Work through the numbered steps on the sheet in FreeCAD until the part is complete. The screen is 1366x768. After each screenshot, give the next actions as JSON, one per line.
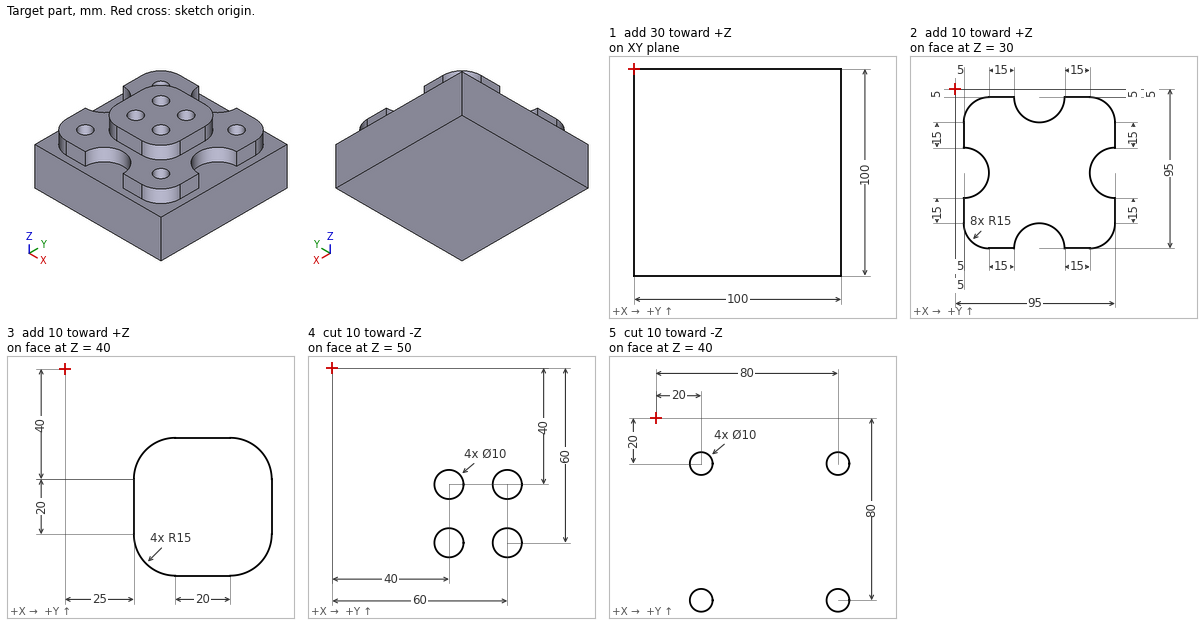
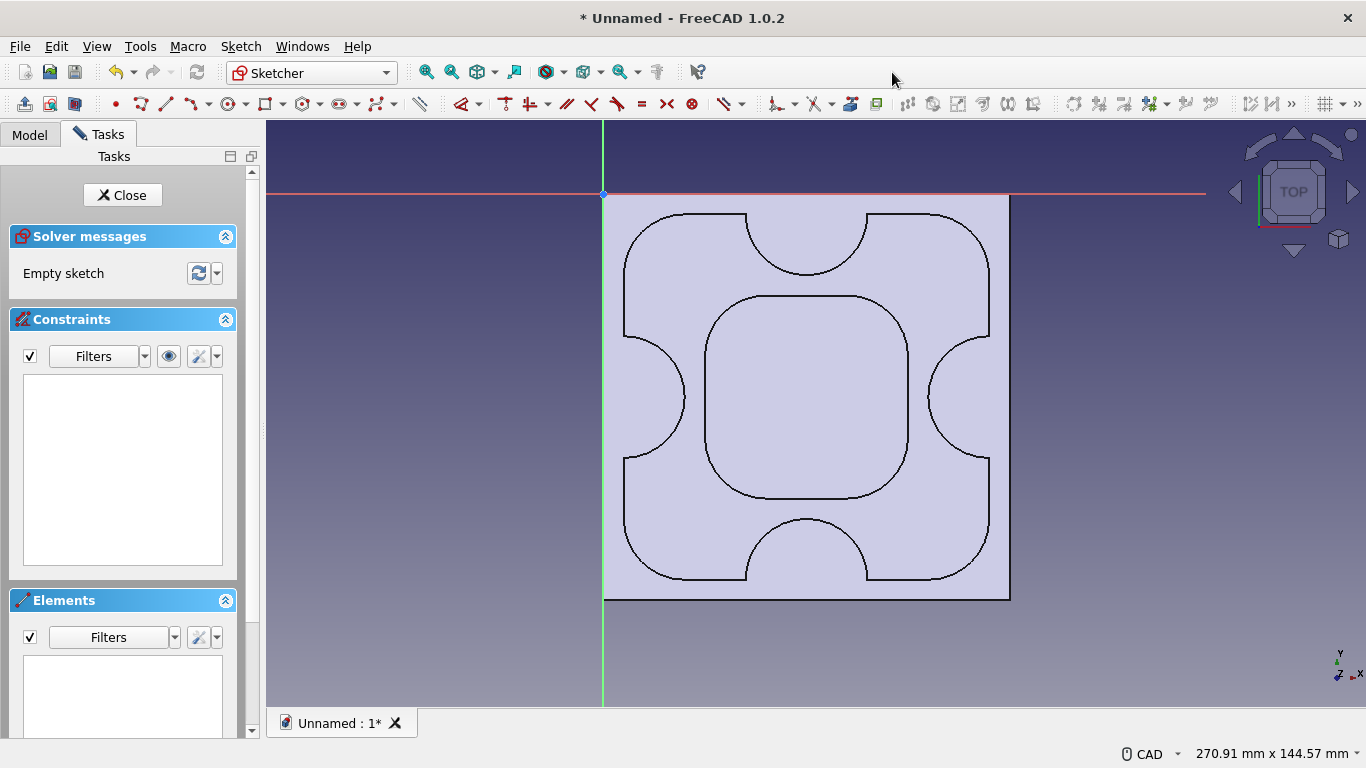
{"action": "scroll", "coordinate": [711, 148], "scroll_direction": "up", "scroll_amount": 2}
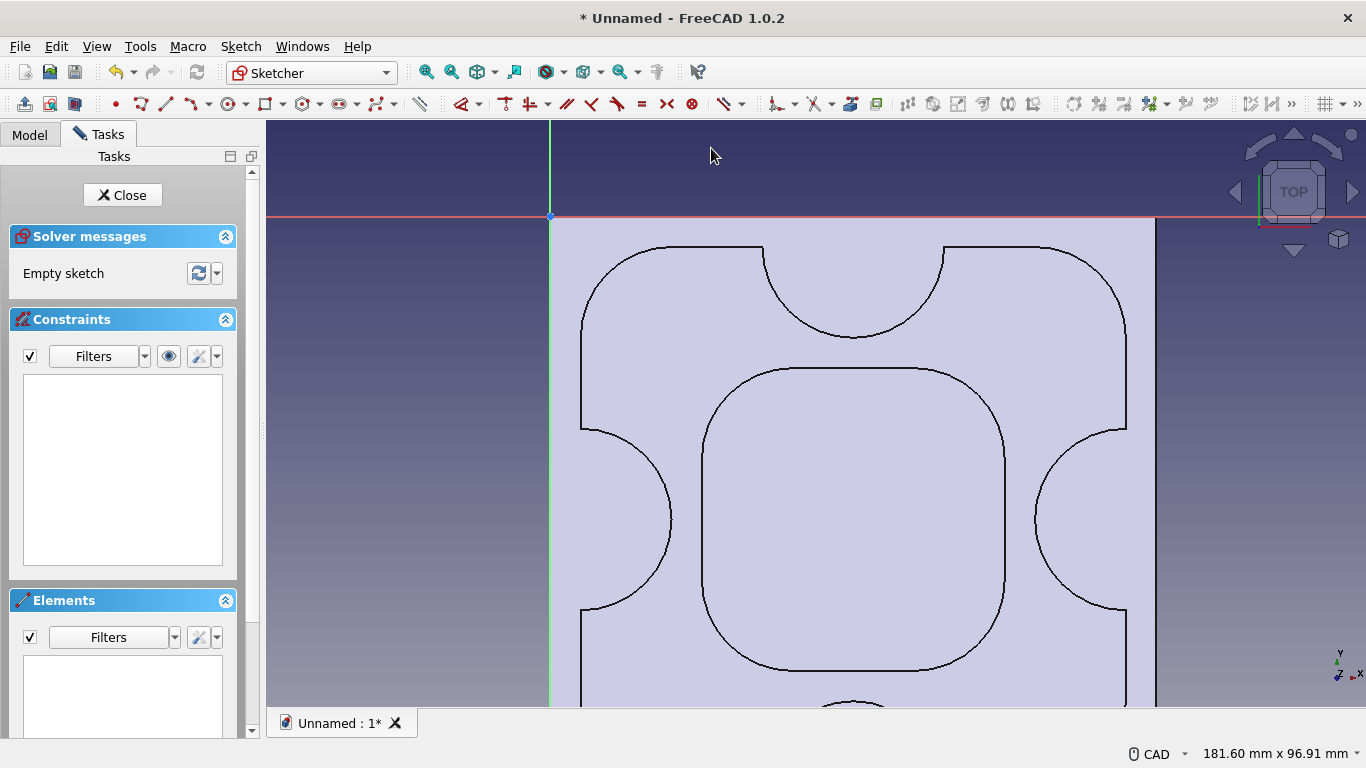
{"action": "left_click", "coordinate": [228, 104]}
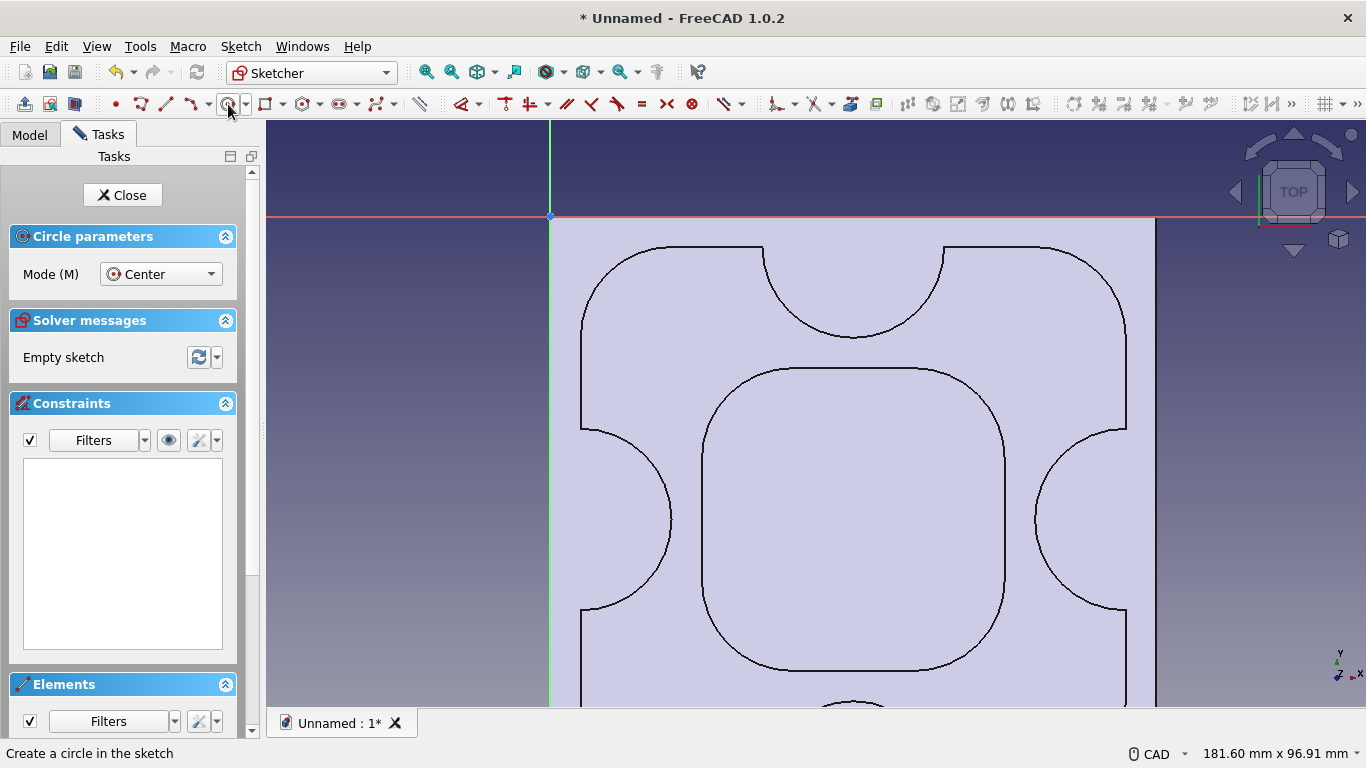
{"action": "left_click", "coordinate": [793, 459]}
{"action": "mouse_move", "coordinate": [814, 438]}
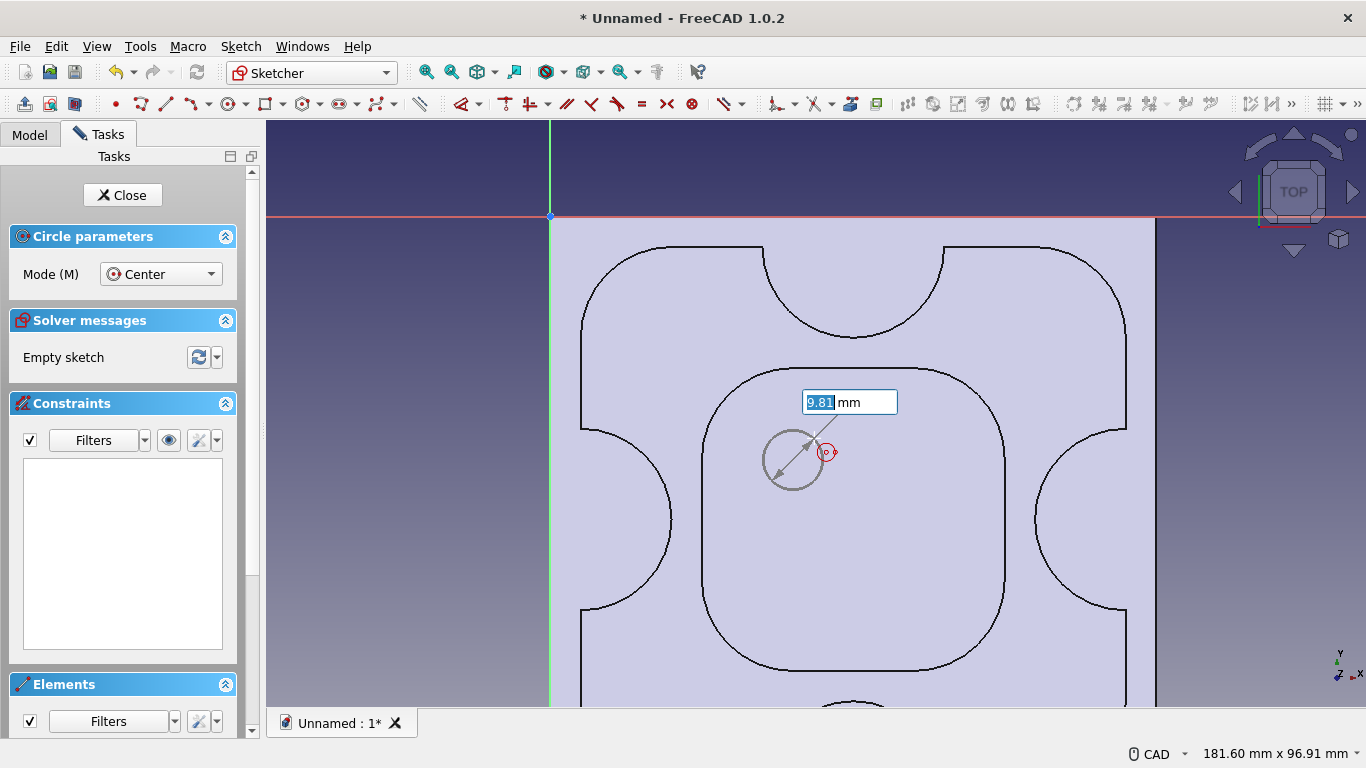
{"action": "type", "text": "10"}
{"action": "key", "text": "Return"}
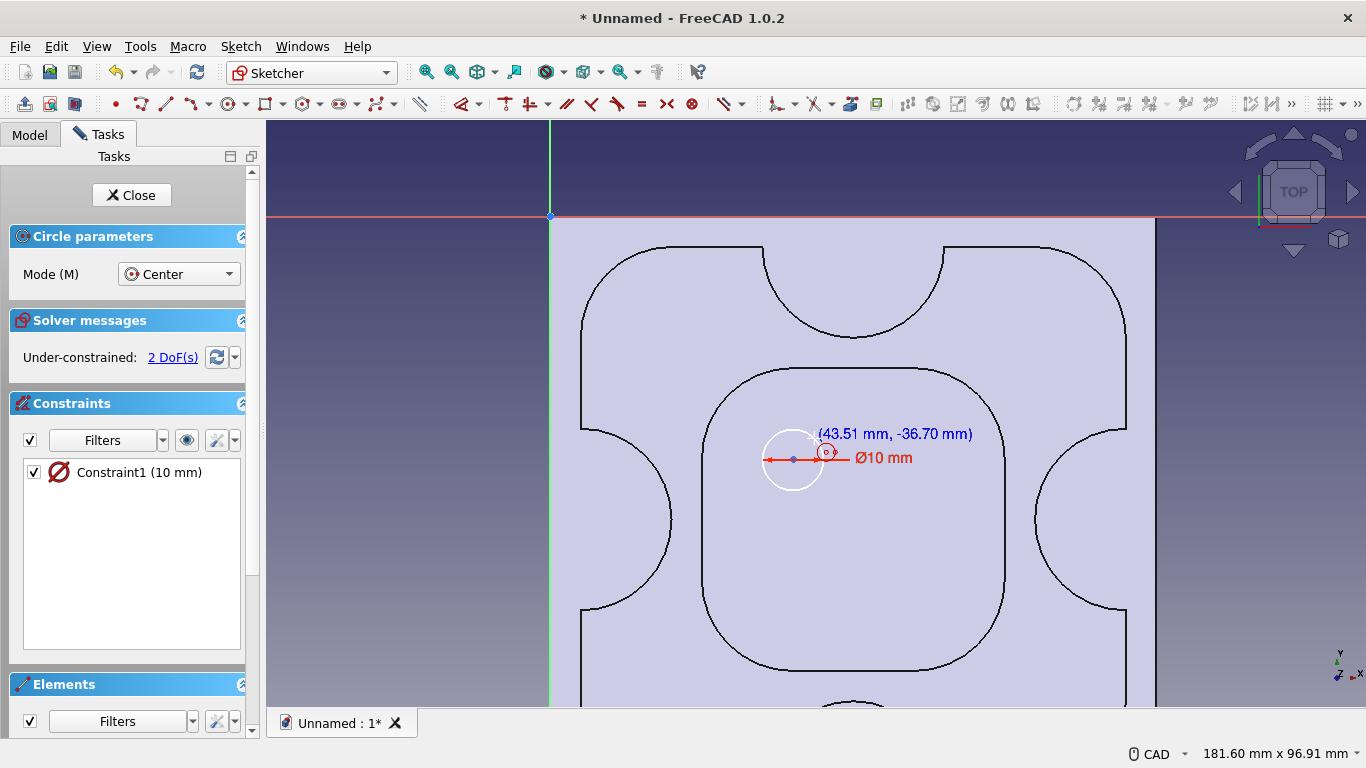
{"action": "left_click", "coordinate": [914, 459]}
{"action": "mouse_move", "coordinate": [935, 438]}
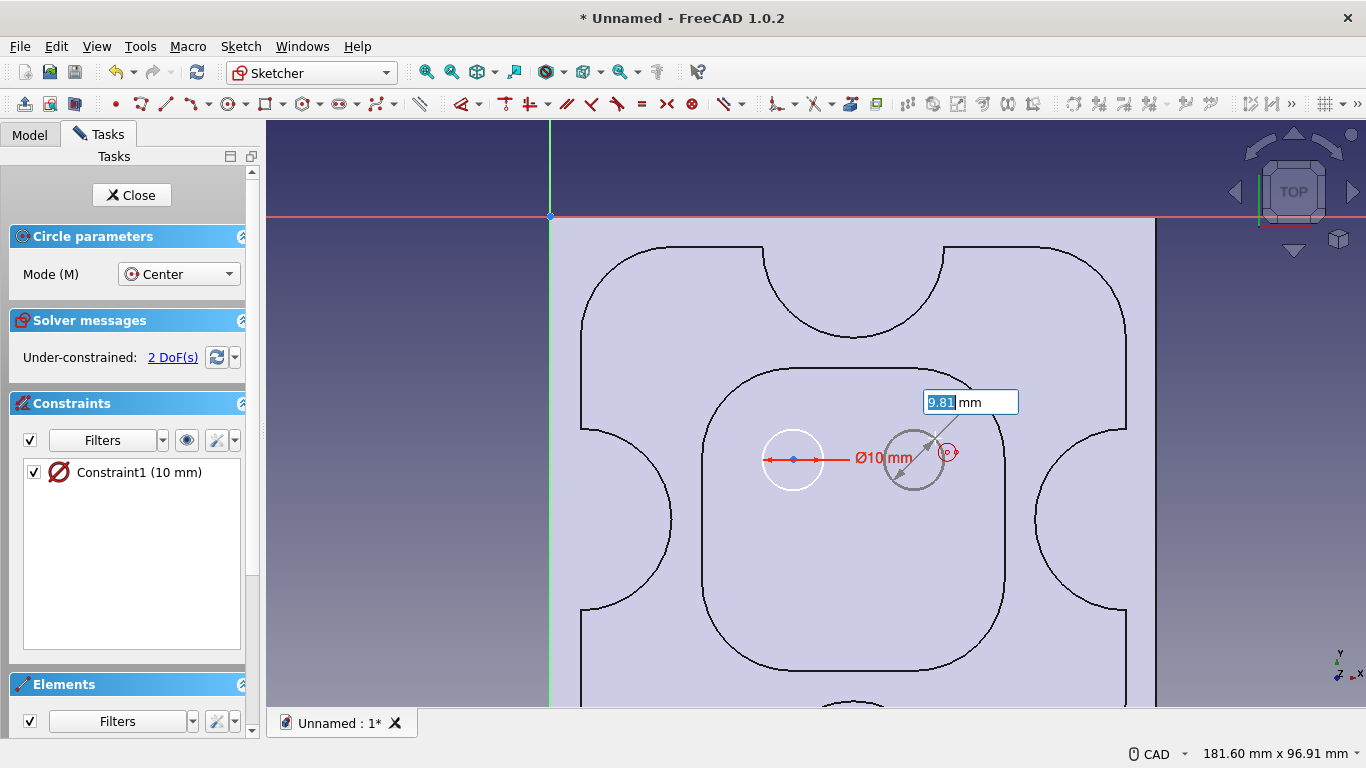
{"action": "type", "text": "10"}
{"action": "key", "text": "Return"}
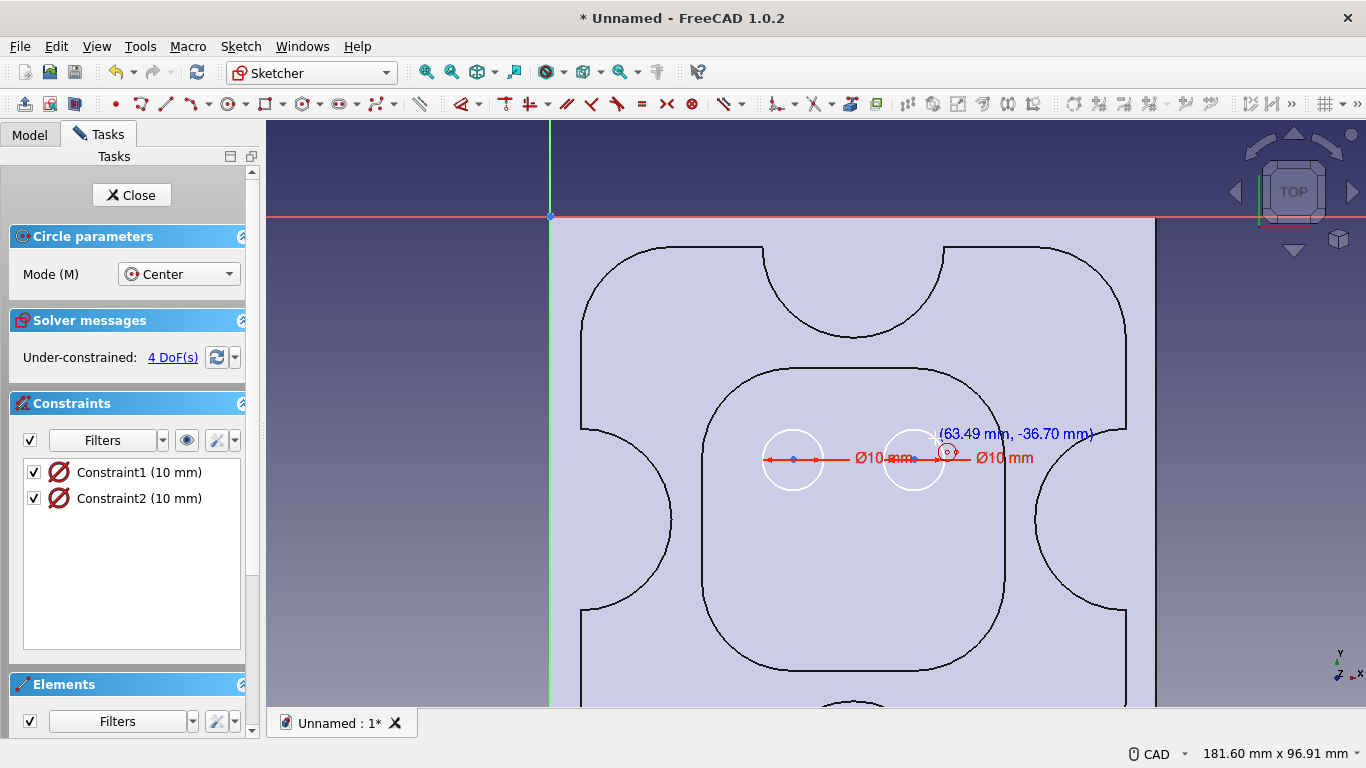
{"action": "left_click", "coordinate": [914, 580]}
{"action": "mouse_move", "coordinate": [935, 559]}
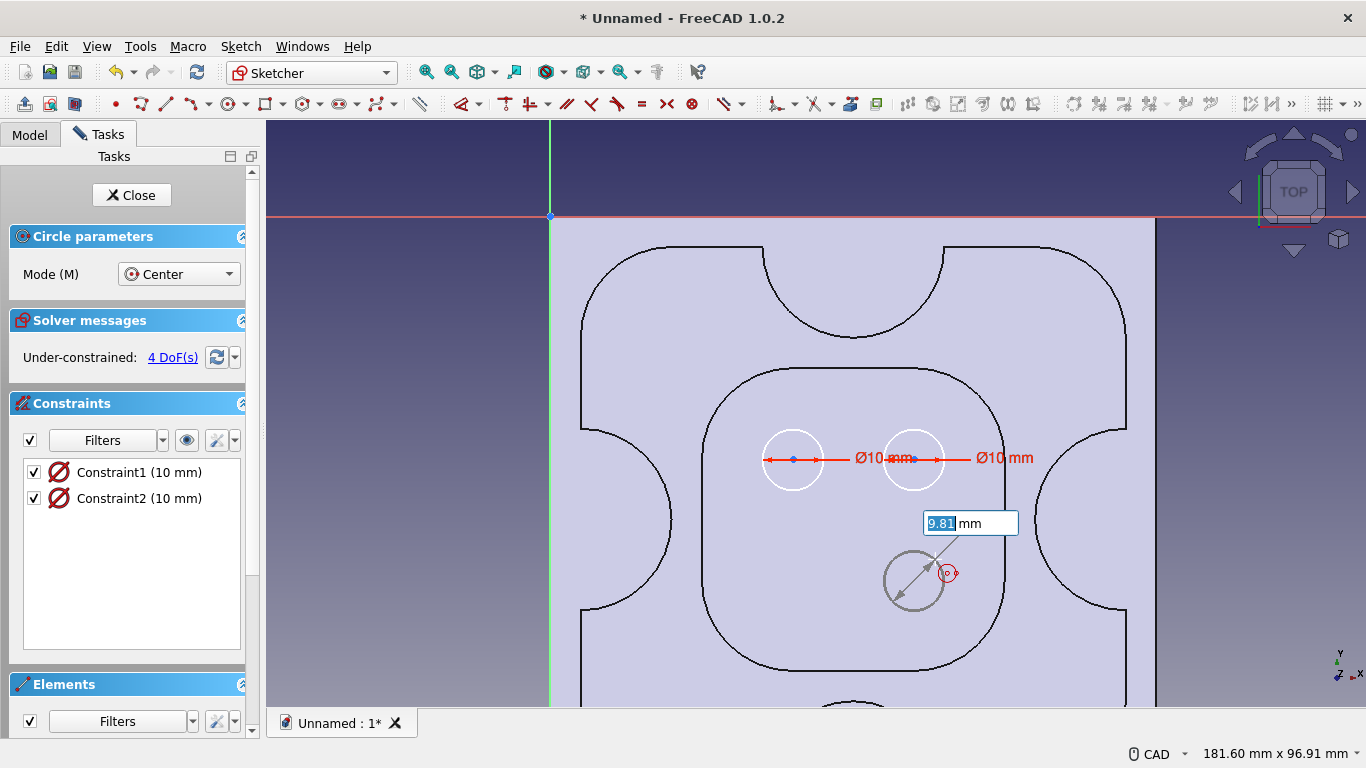
{"action": "type", "text": "10"}
{"action": "key", "text": "Return"}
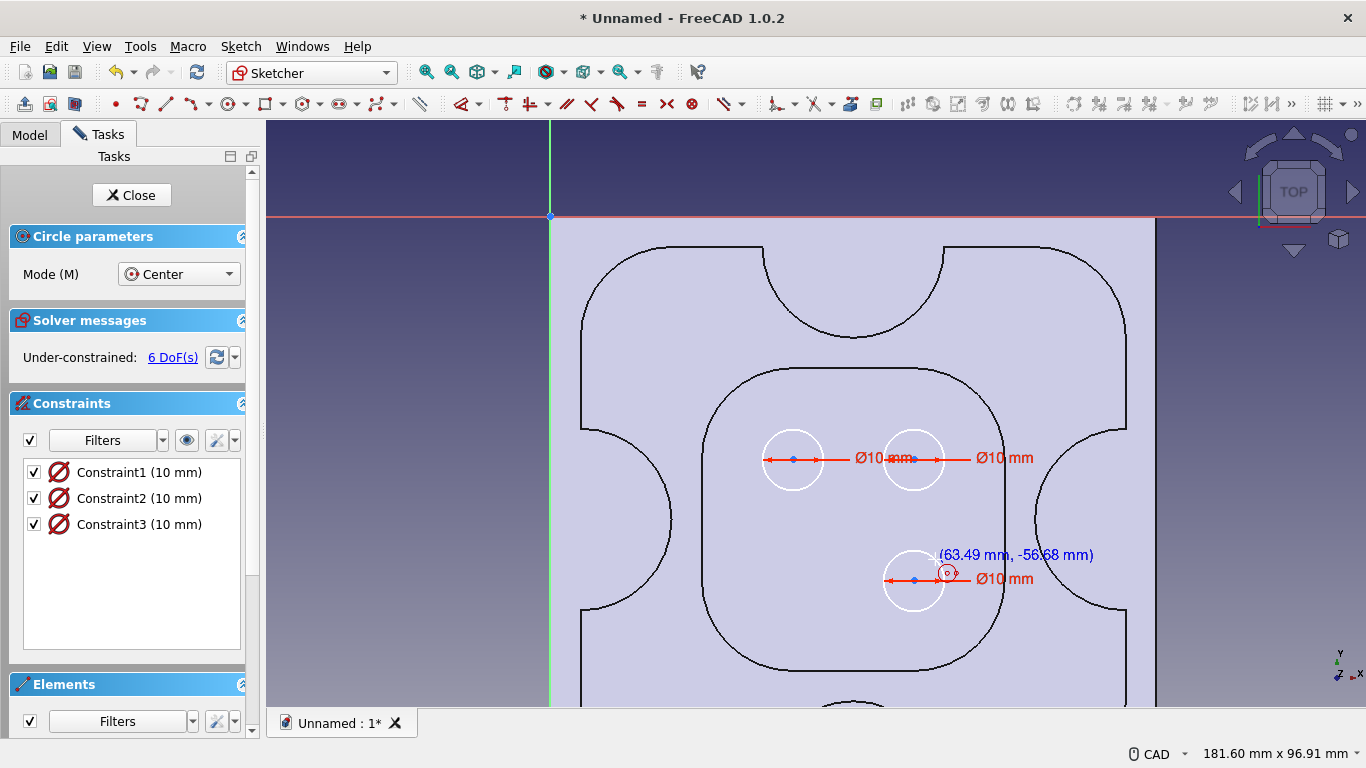
{"action": "left_click", "coordinate": [793, 580]}
{"action": "mouse_move", "coordinate": [814, 559]}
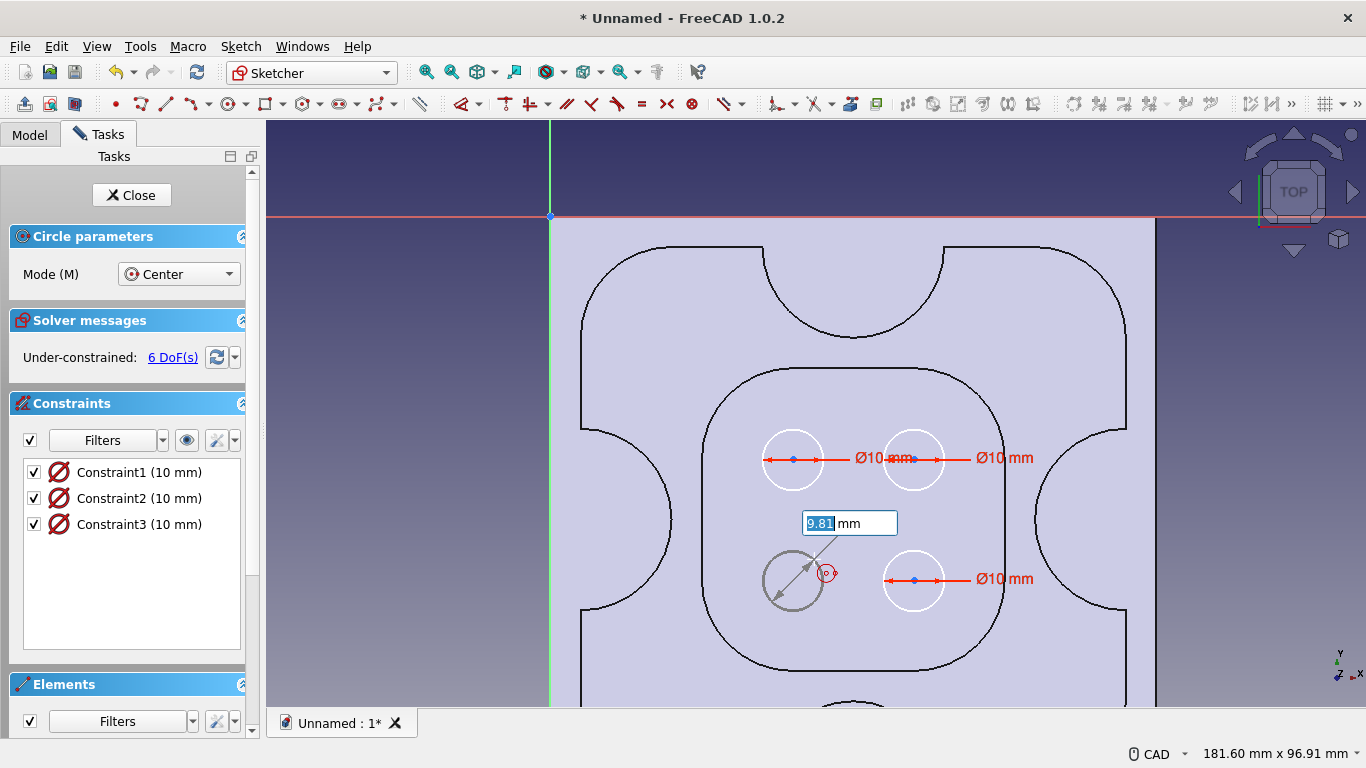
{"action": "type", "text": "10"}
{"action": "key", "text": "Return"}
{"action": "key", "text": "Escape"}